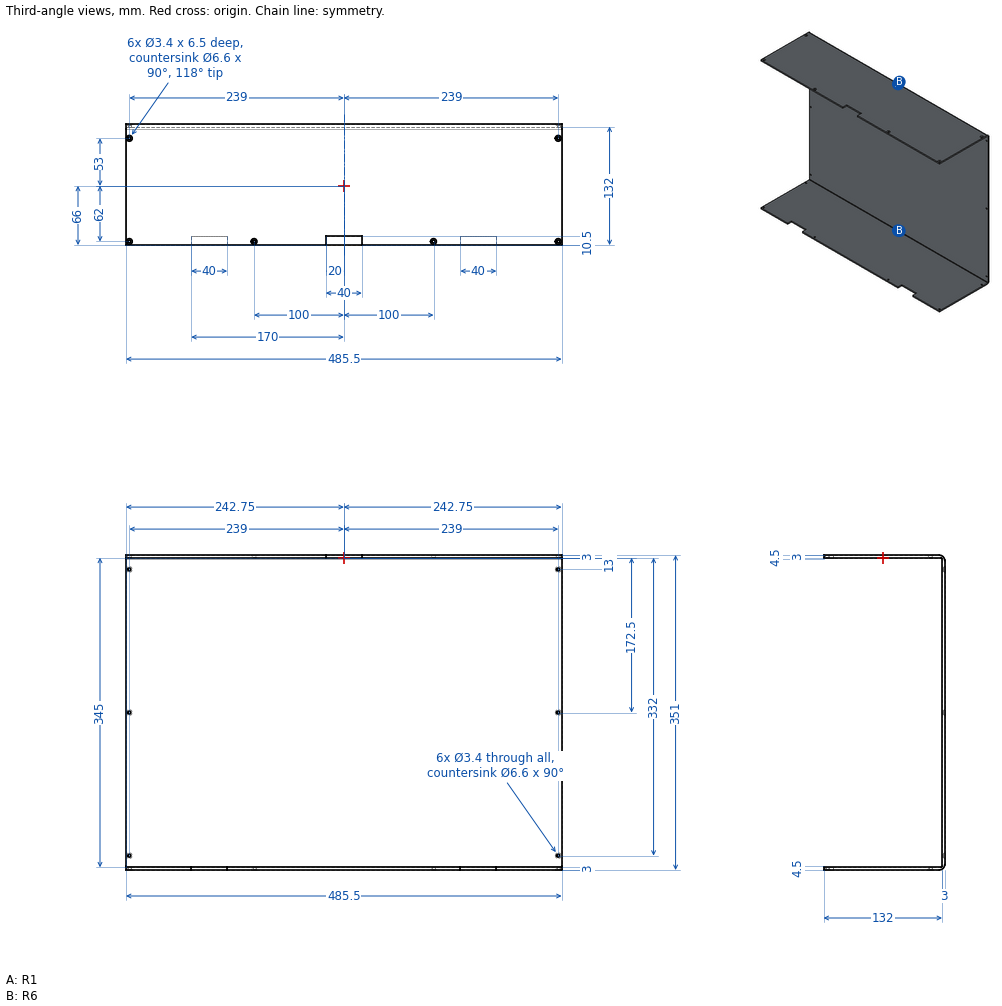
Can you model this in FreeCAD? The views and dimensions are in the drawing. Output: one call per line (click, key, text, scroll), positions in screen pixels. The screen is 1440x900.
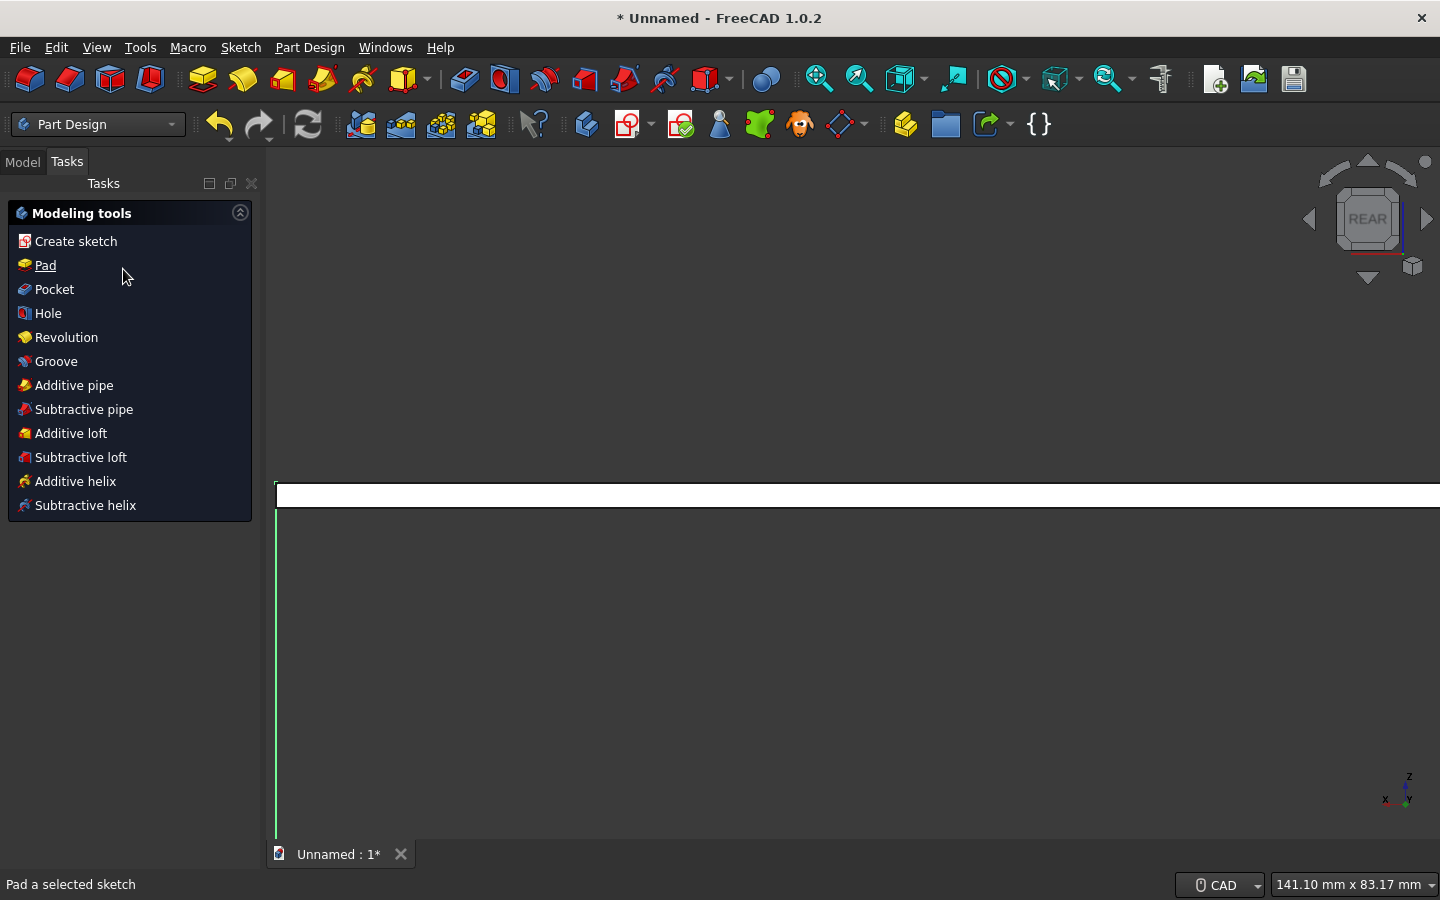
click(204, 80)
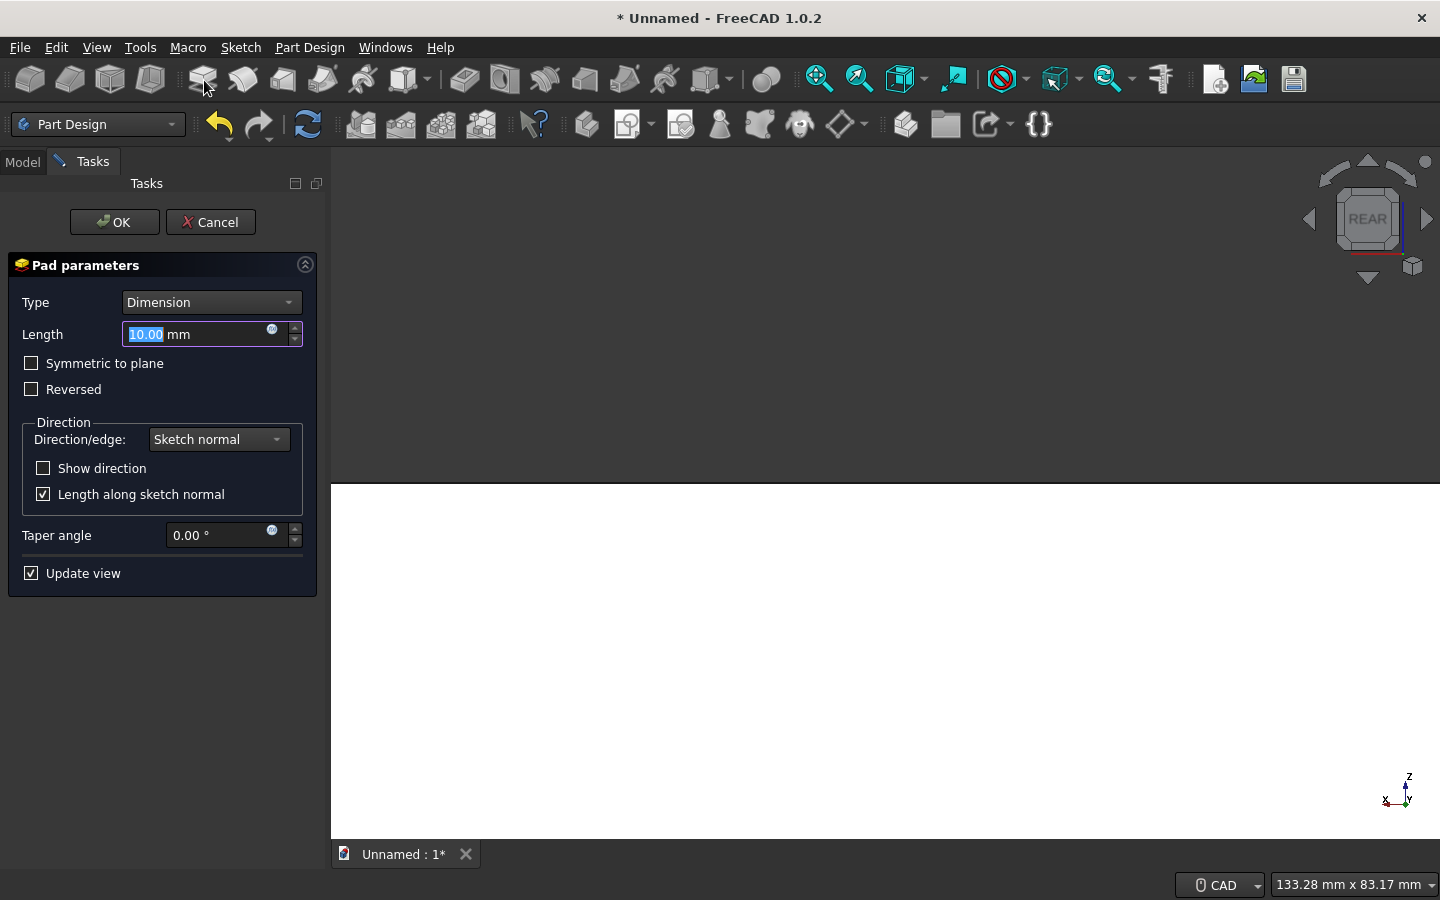
text(3)
key(Tab)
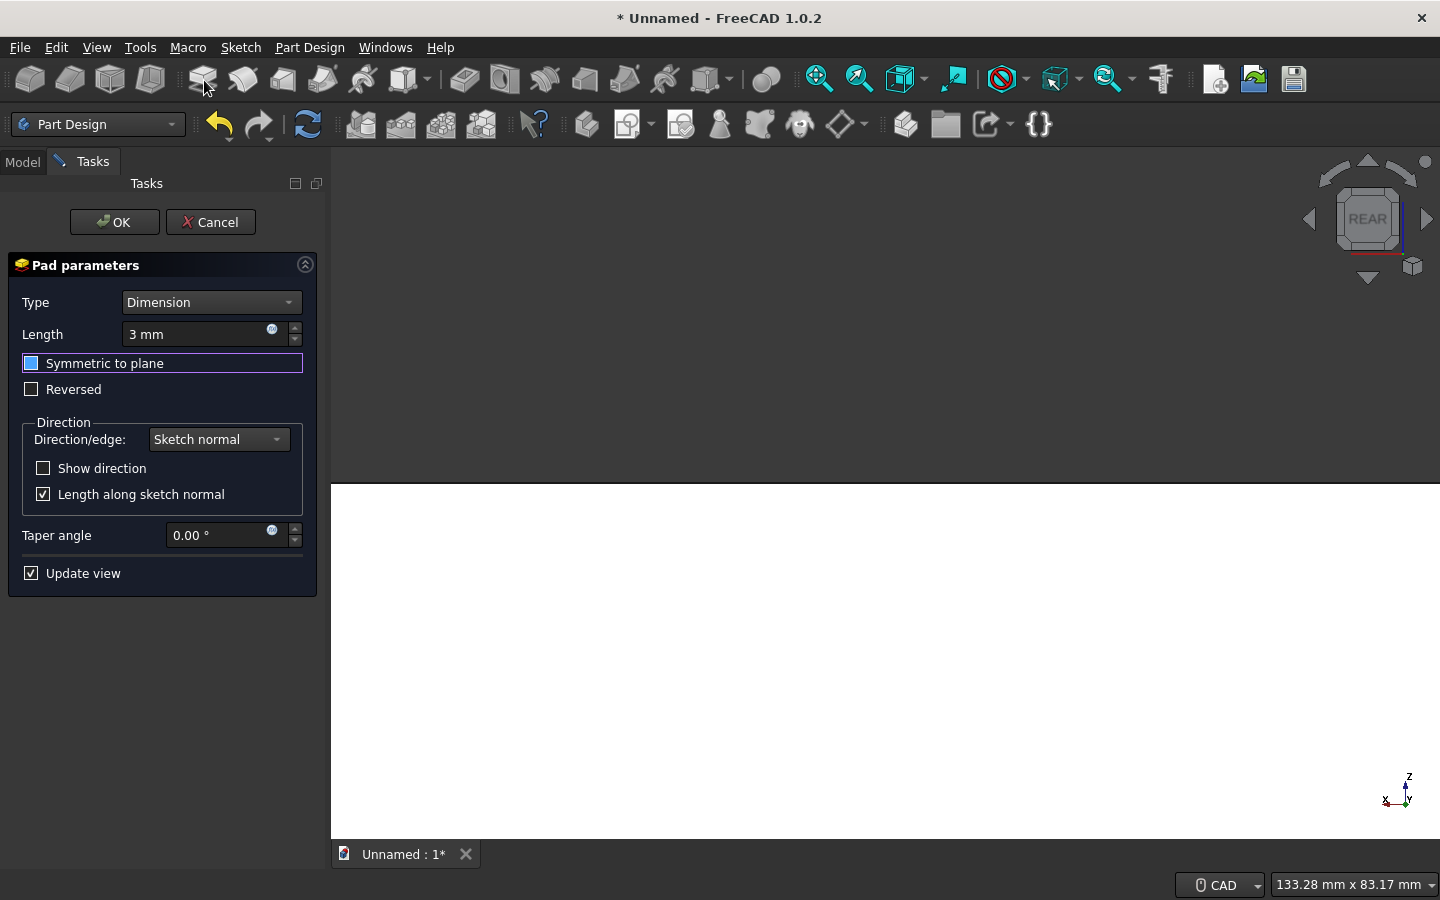
click(115, 222)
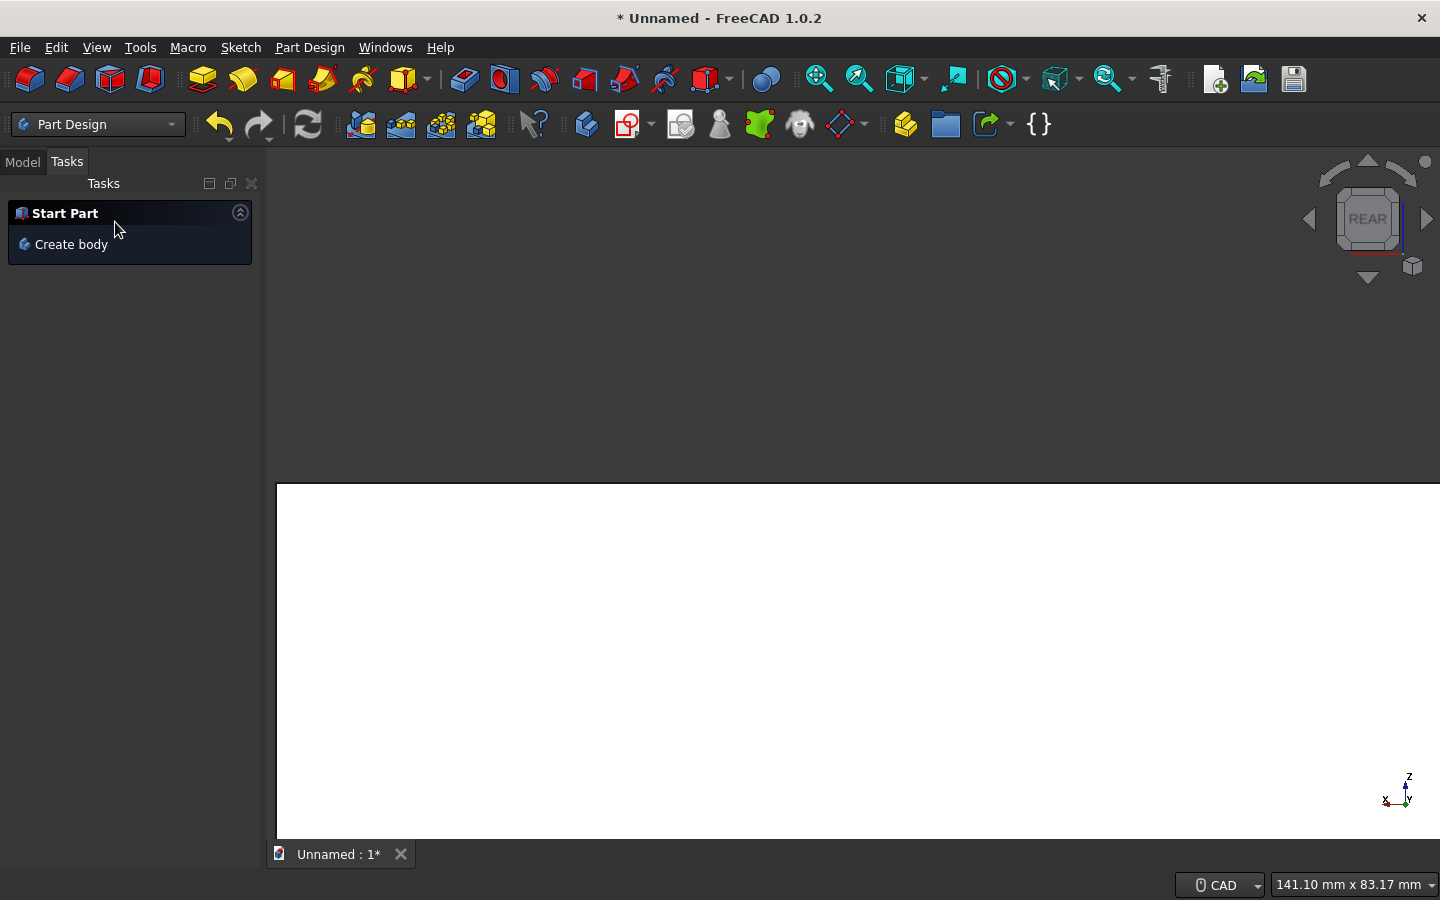
click(820, 80)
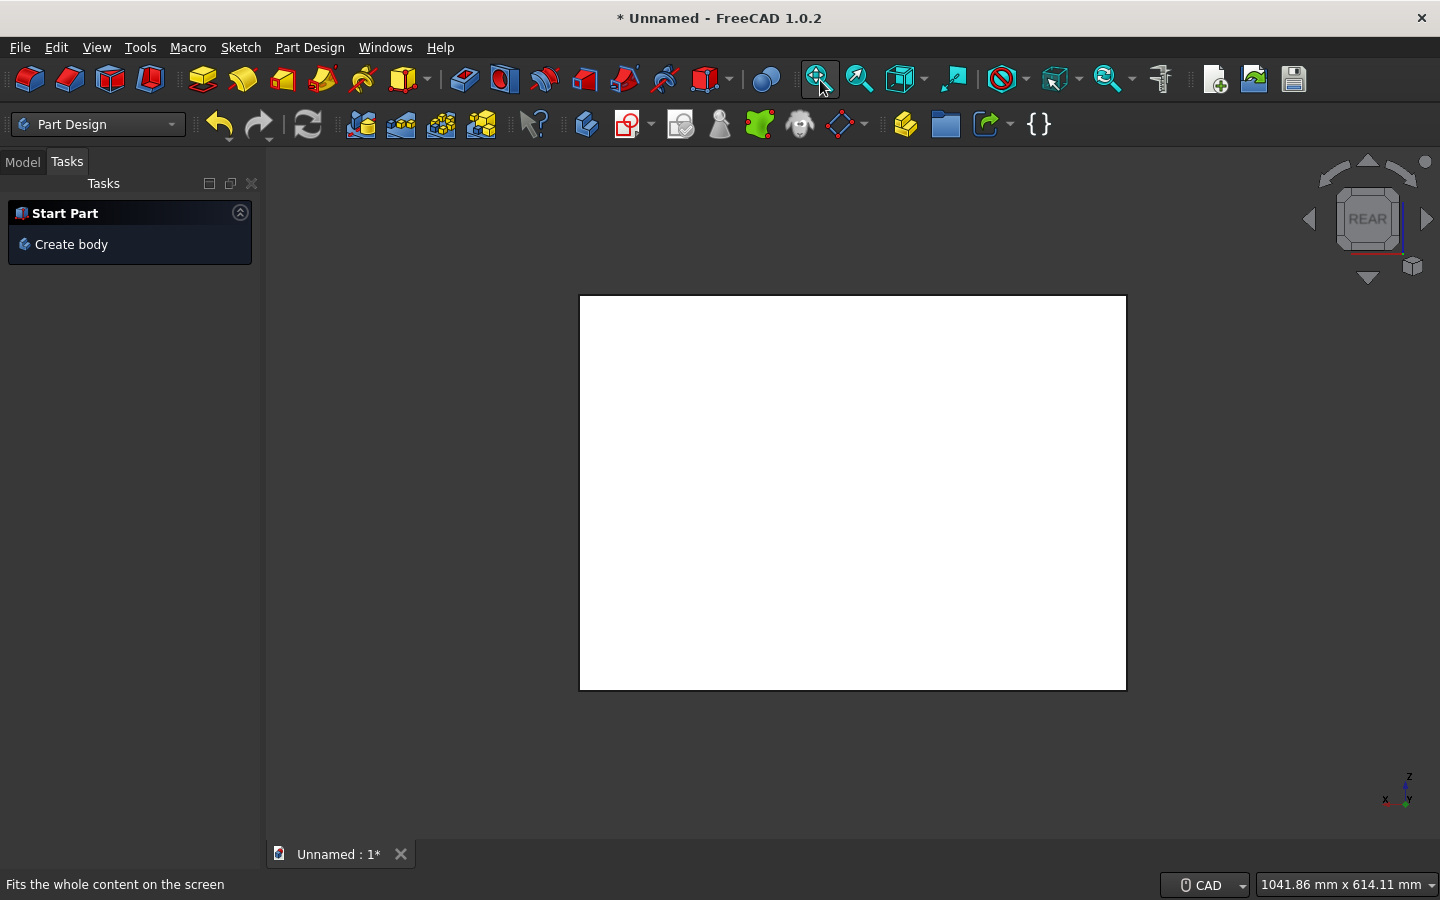
key(0)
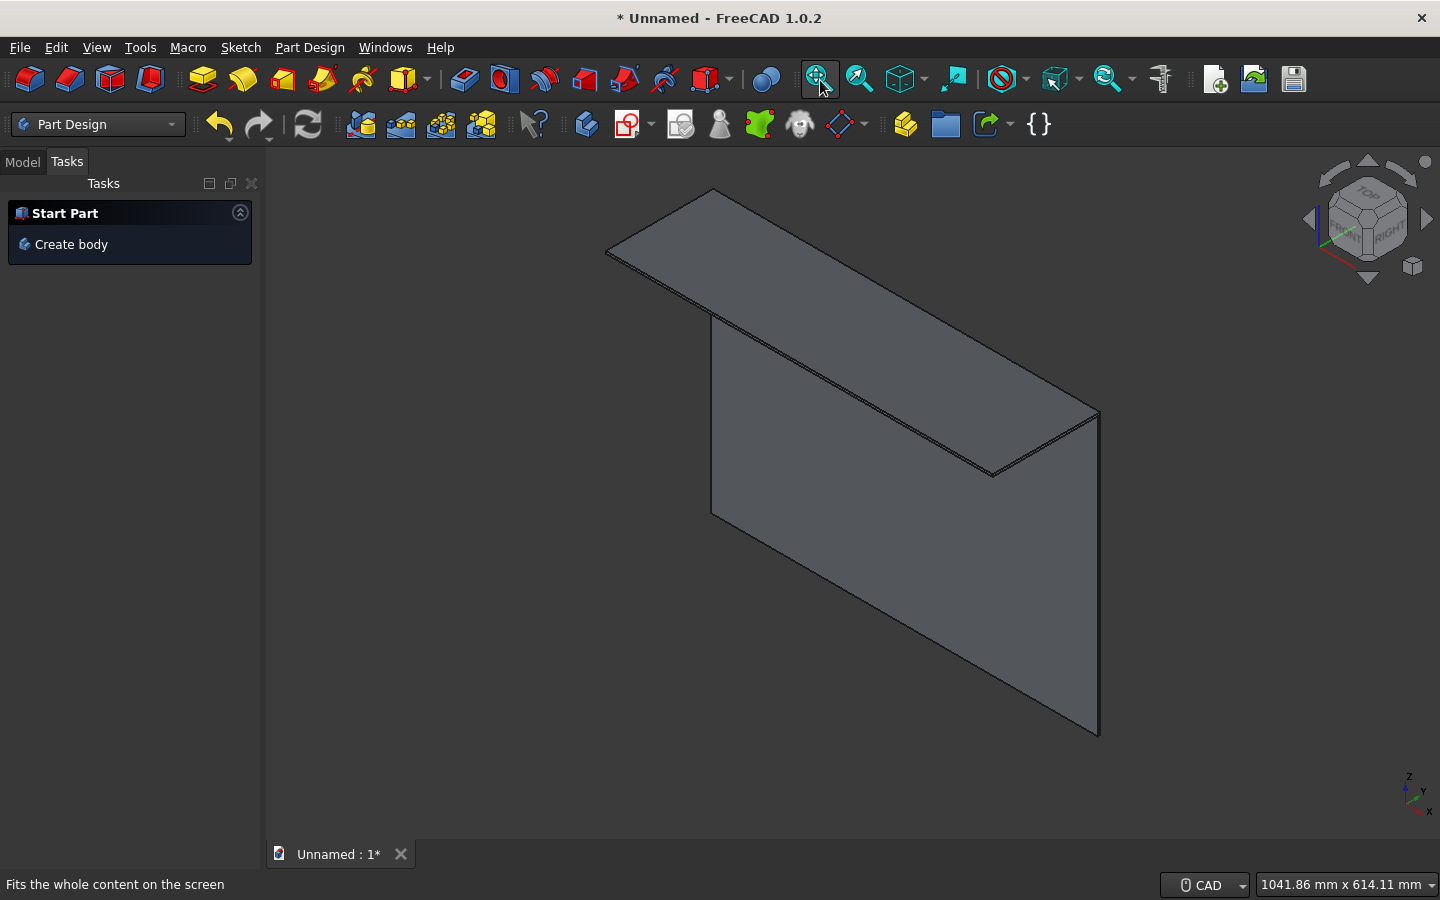
click(904, 464)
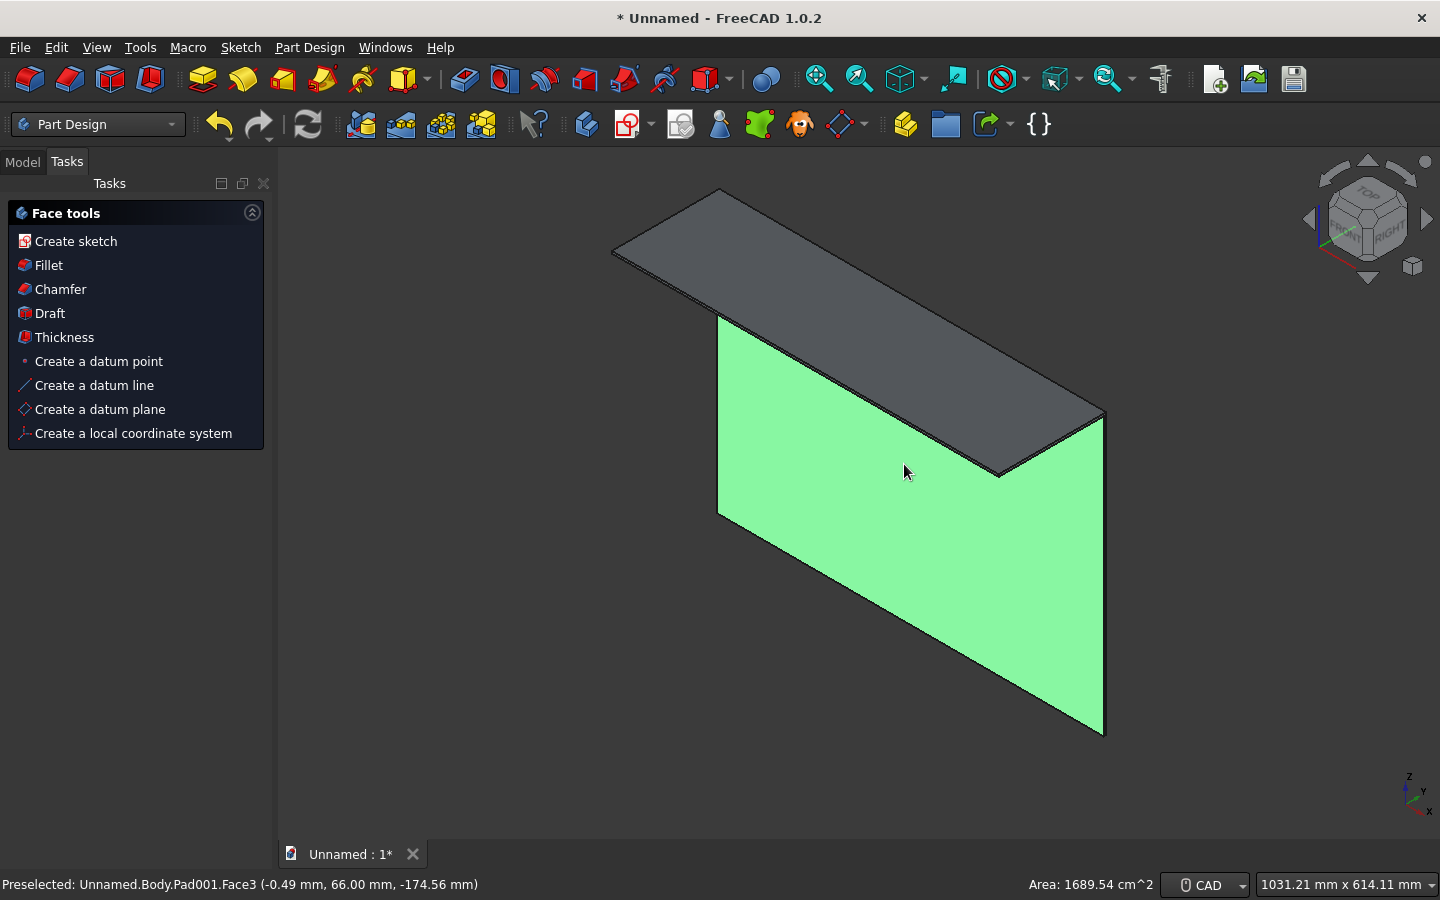
click(628, 124)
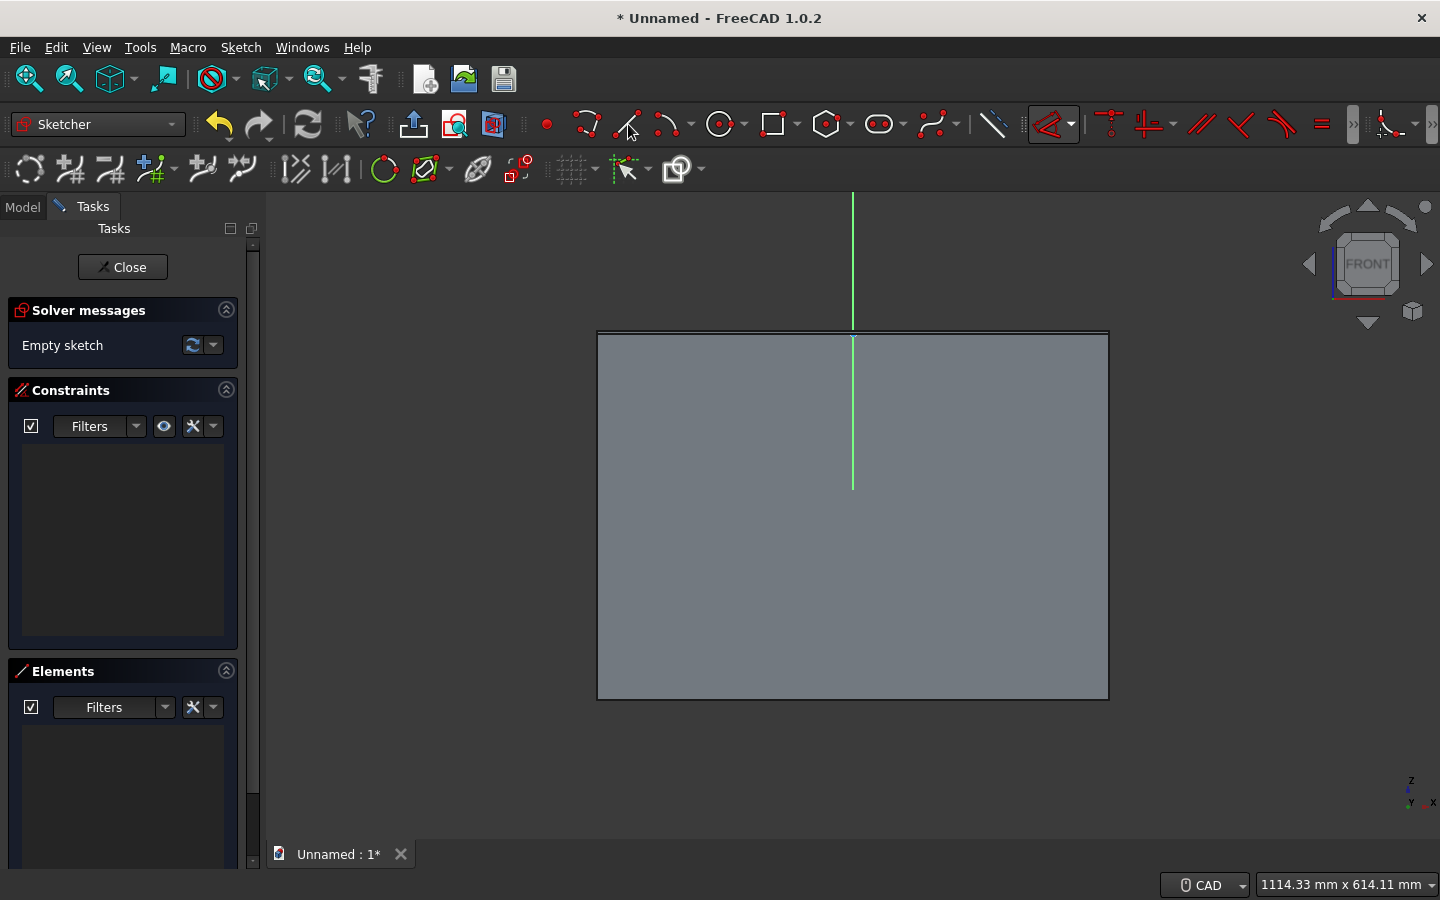
click(774, 124)